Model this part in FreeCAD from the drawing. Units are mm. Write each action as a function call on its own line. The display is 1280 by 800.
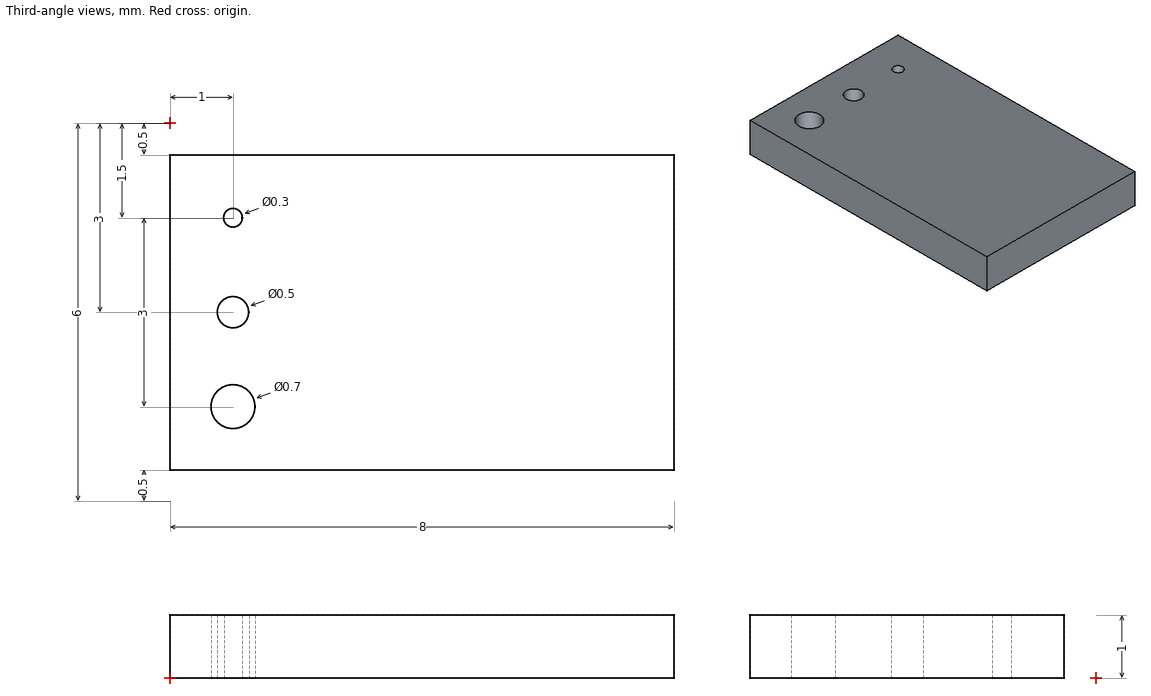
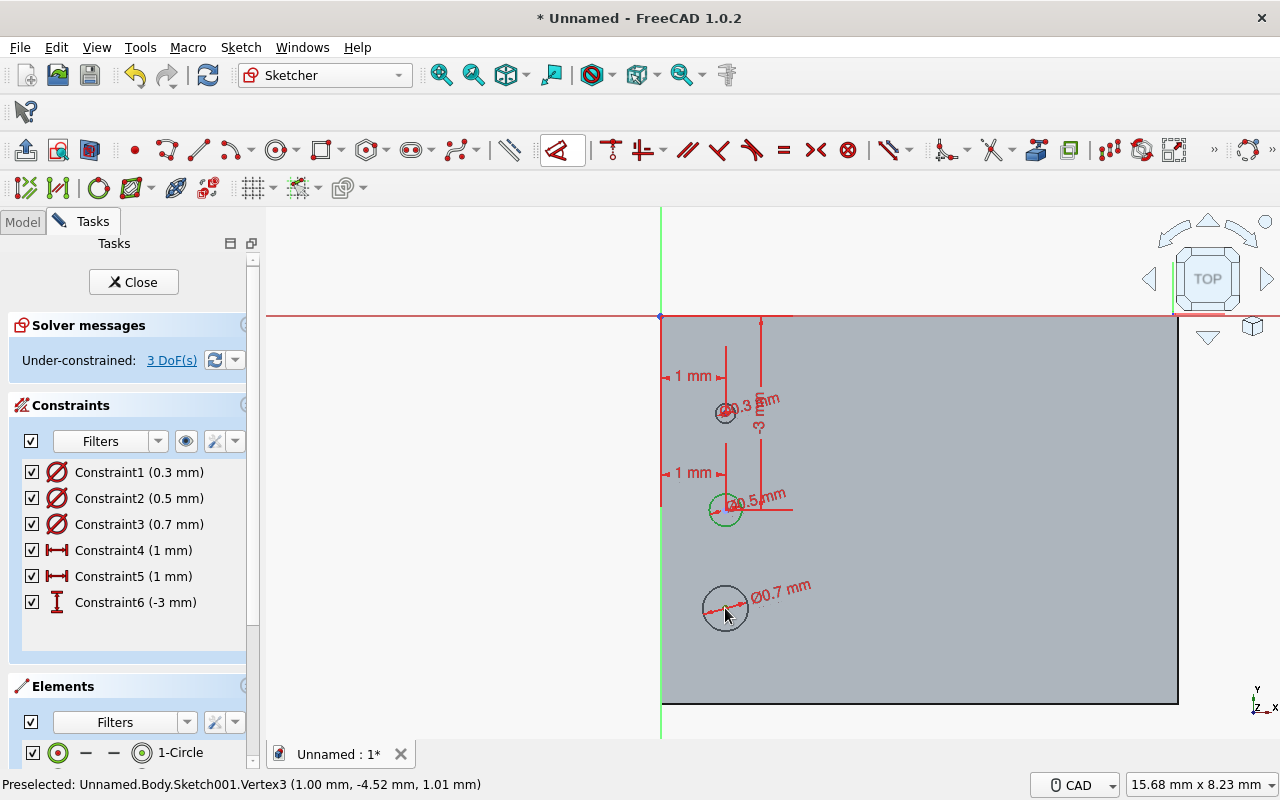
key(l)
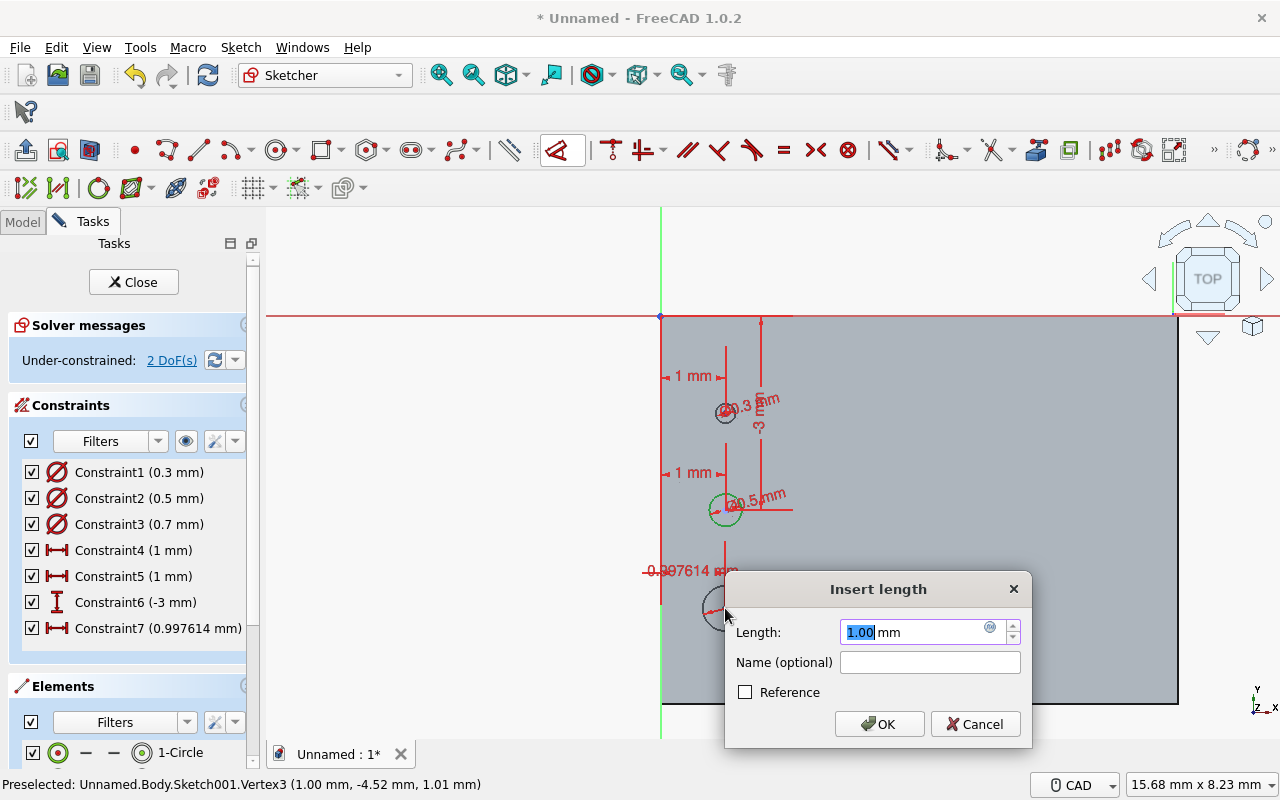
text(1)
key(Return)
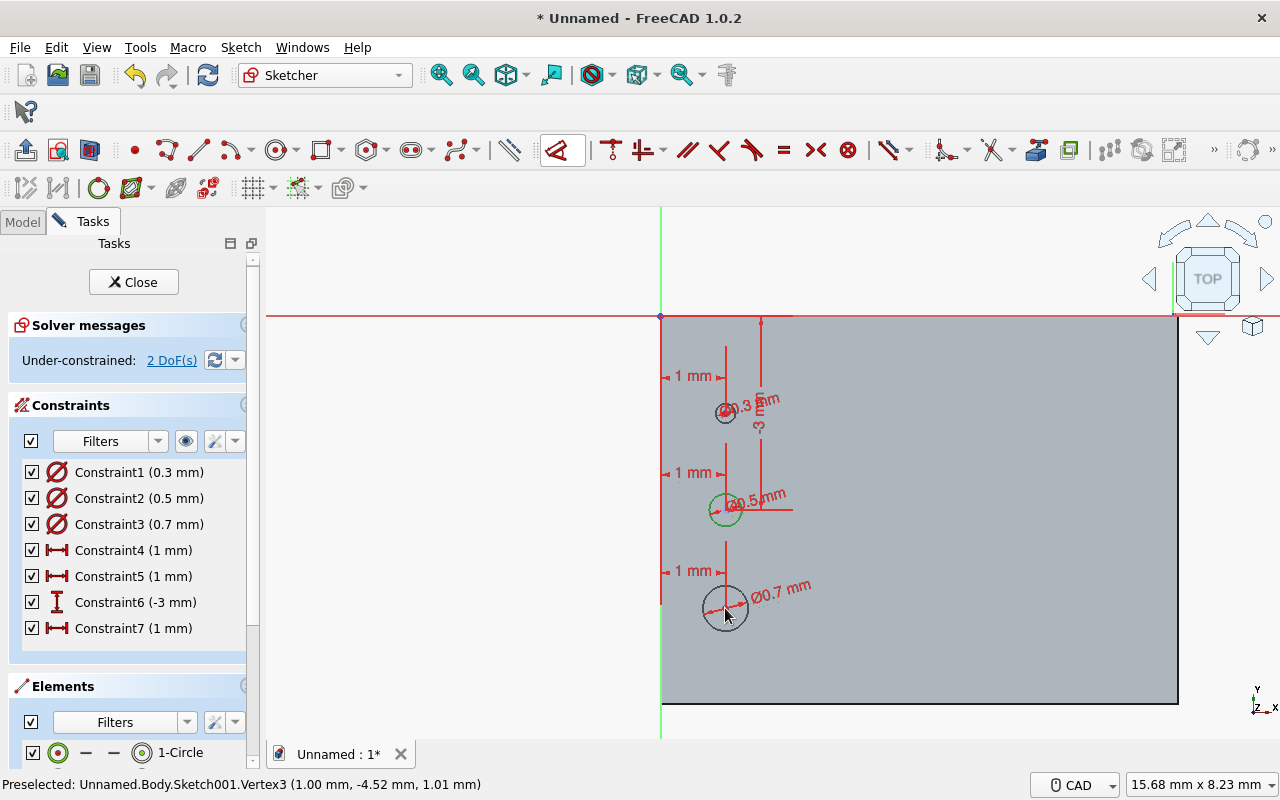
click(726, 414)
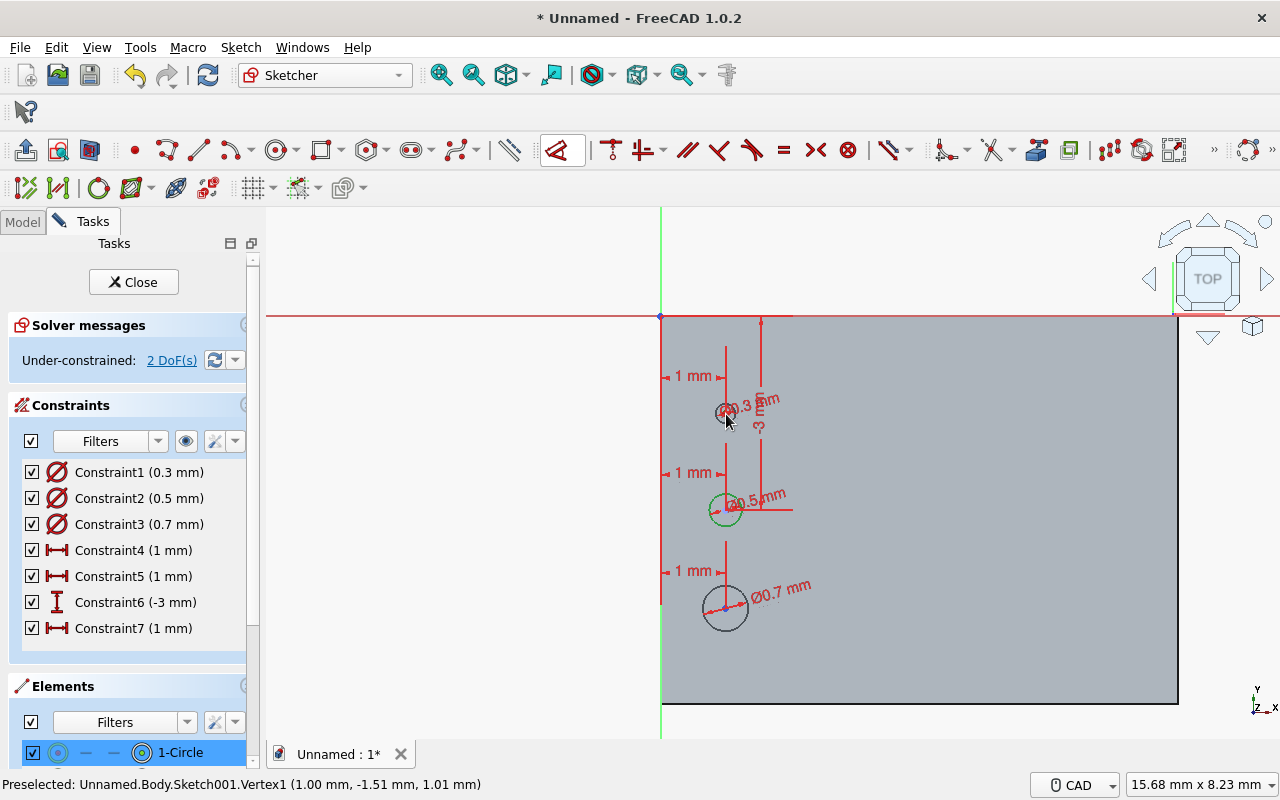
click(726, 608)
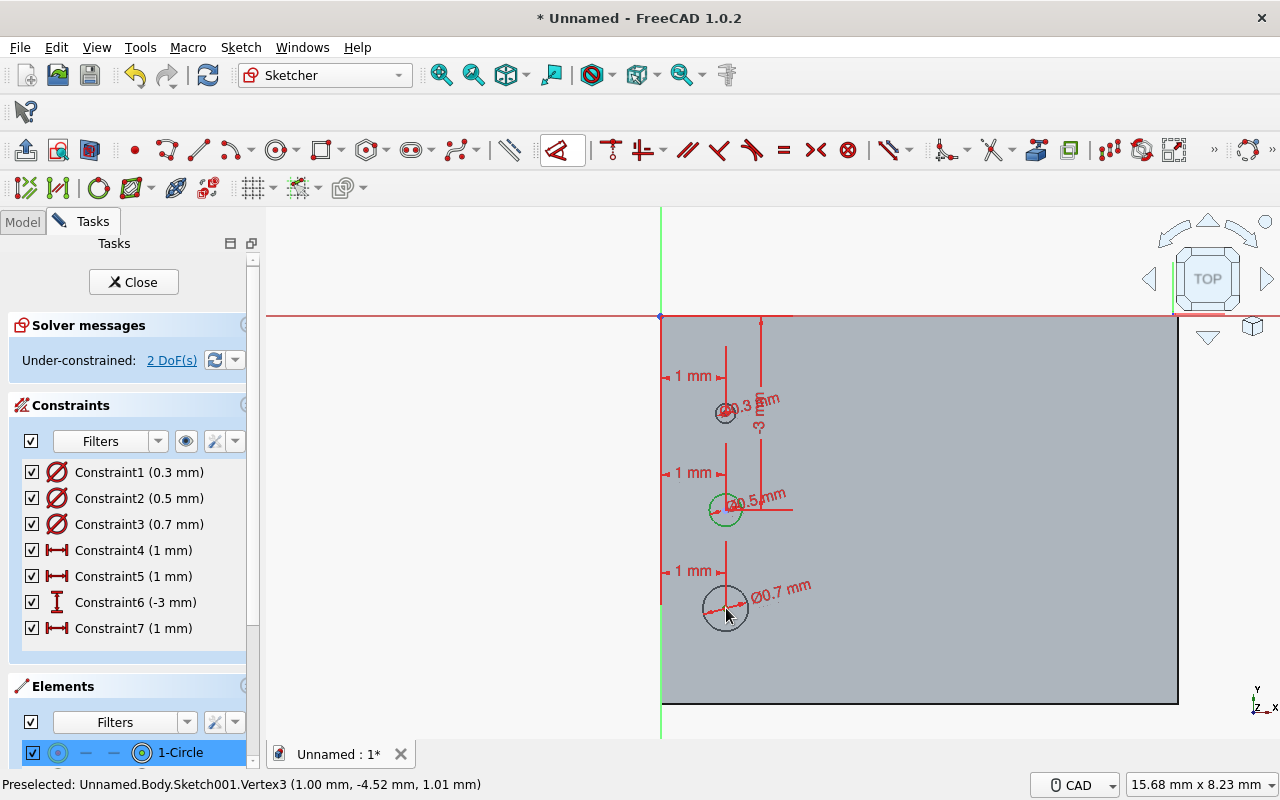
key(i)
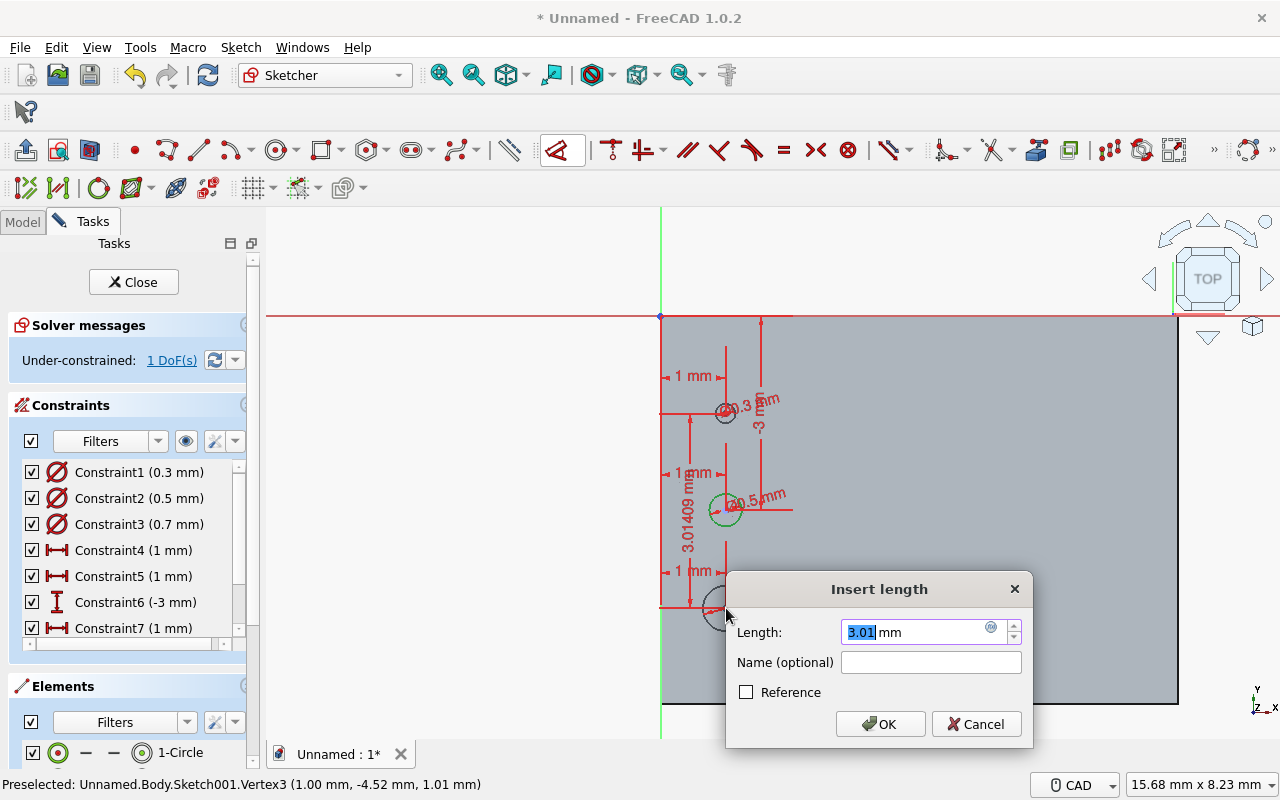
text(3)
key(Return)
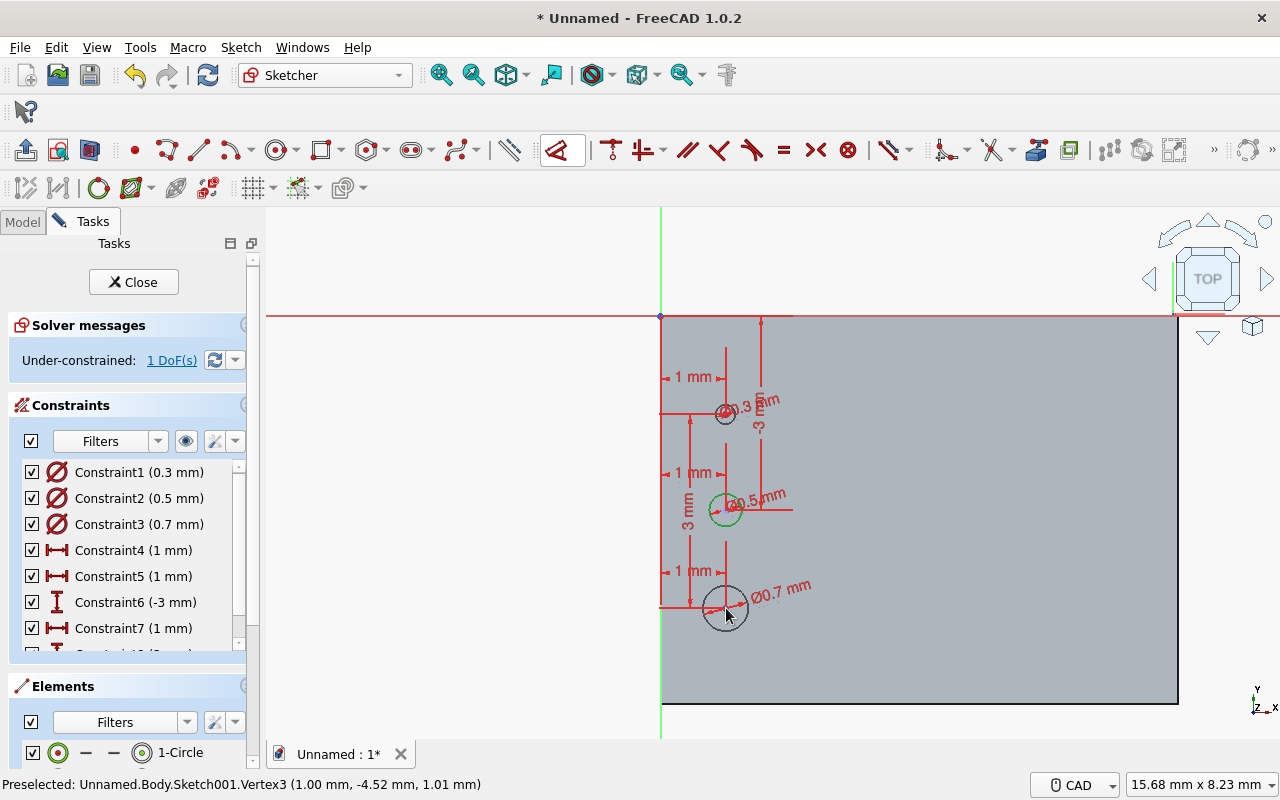
click(726, 414)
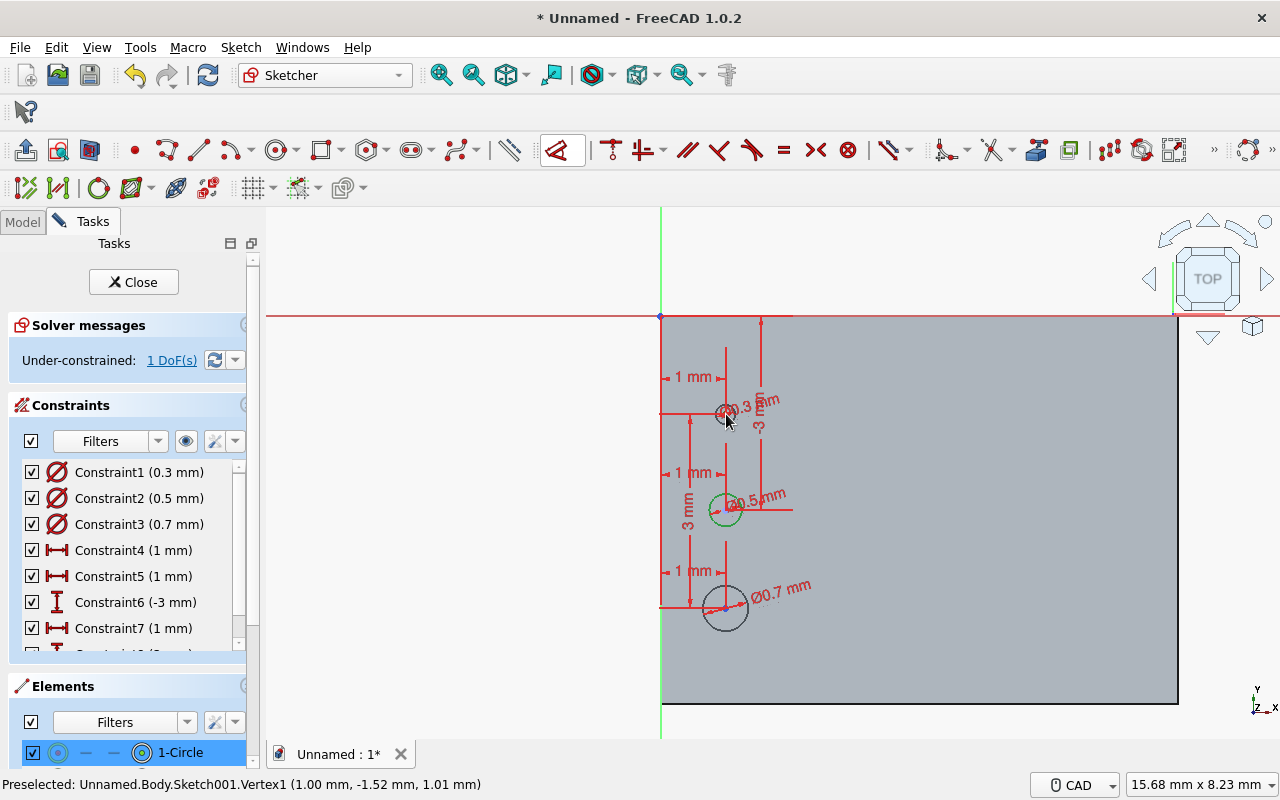
key(i)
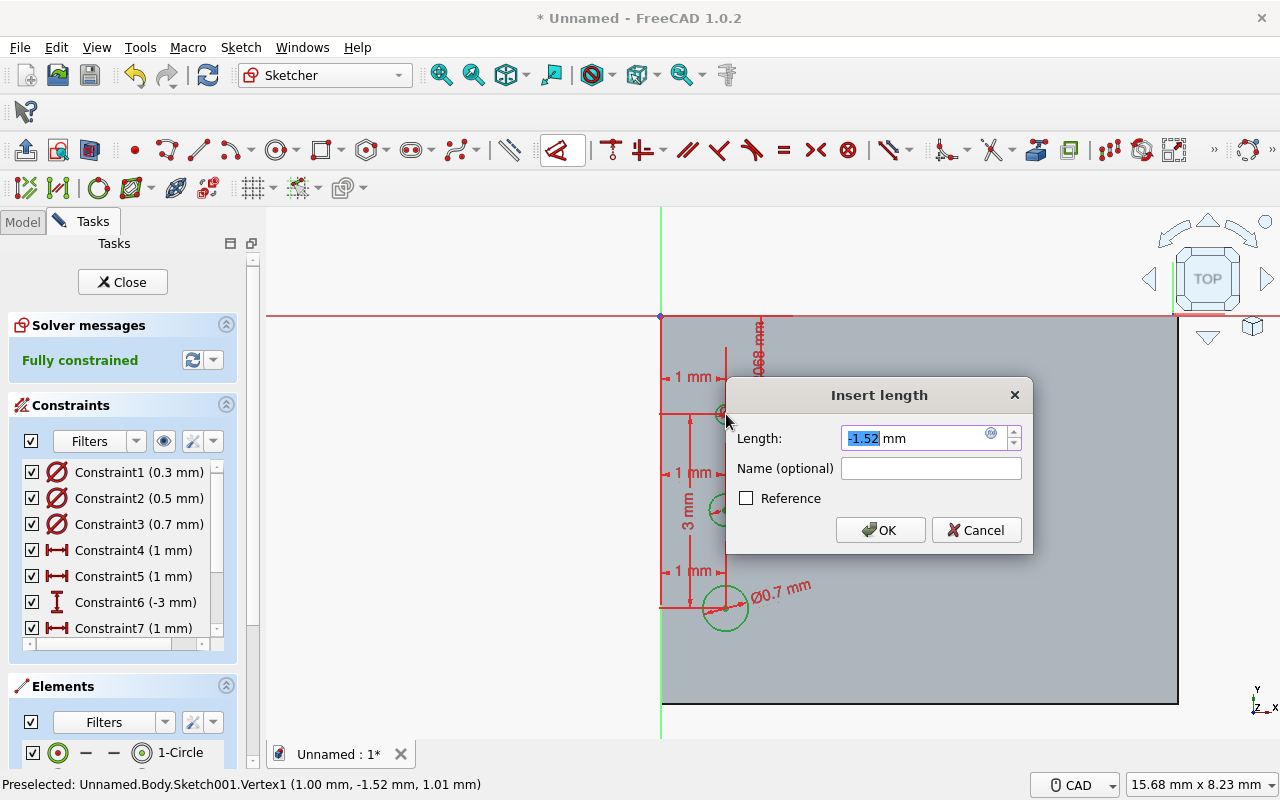
text(-1.5)
key(Return)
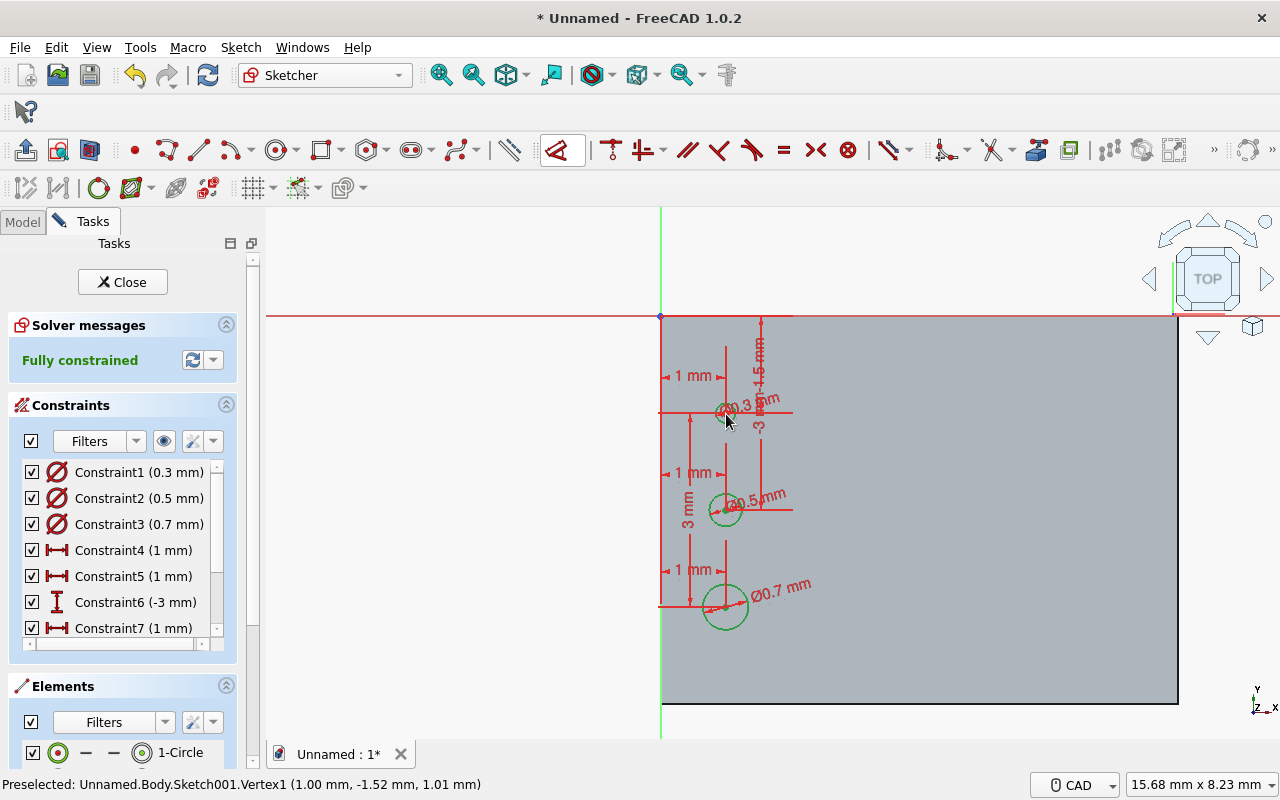
click(123, 282)